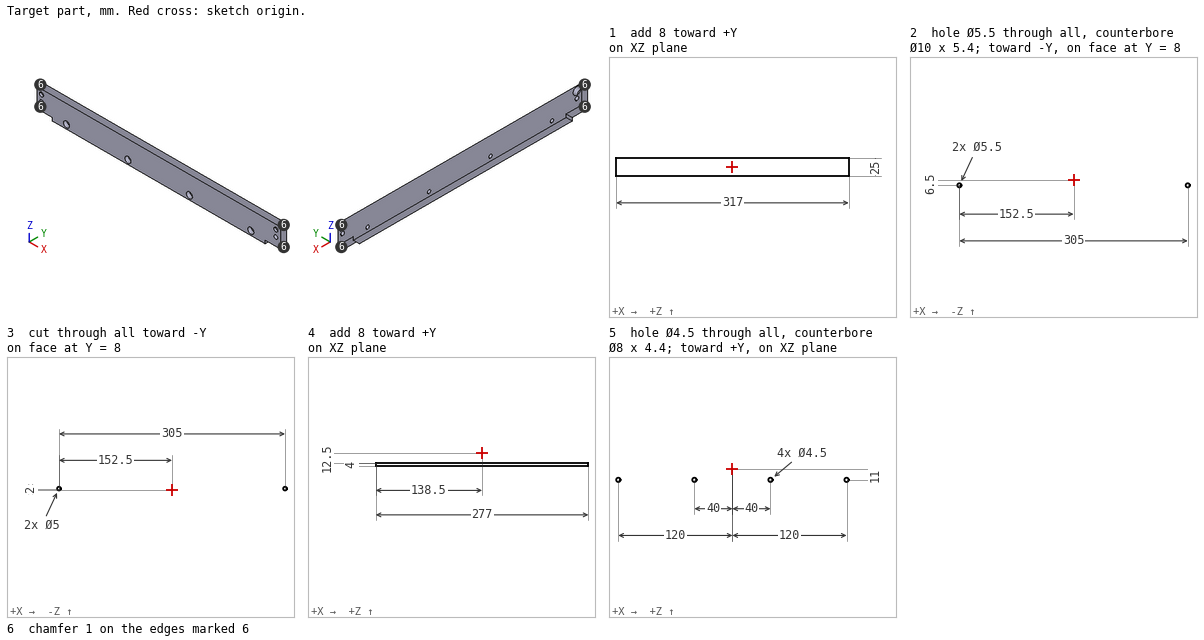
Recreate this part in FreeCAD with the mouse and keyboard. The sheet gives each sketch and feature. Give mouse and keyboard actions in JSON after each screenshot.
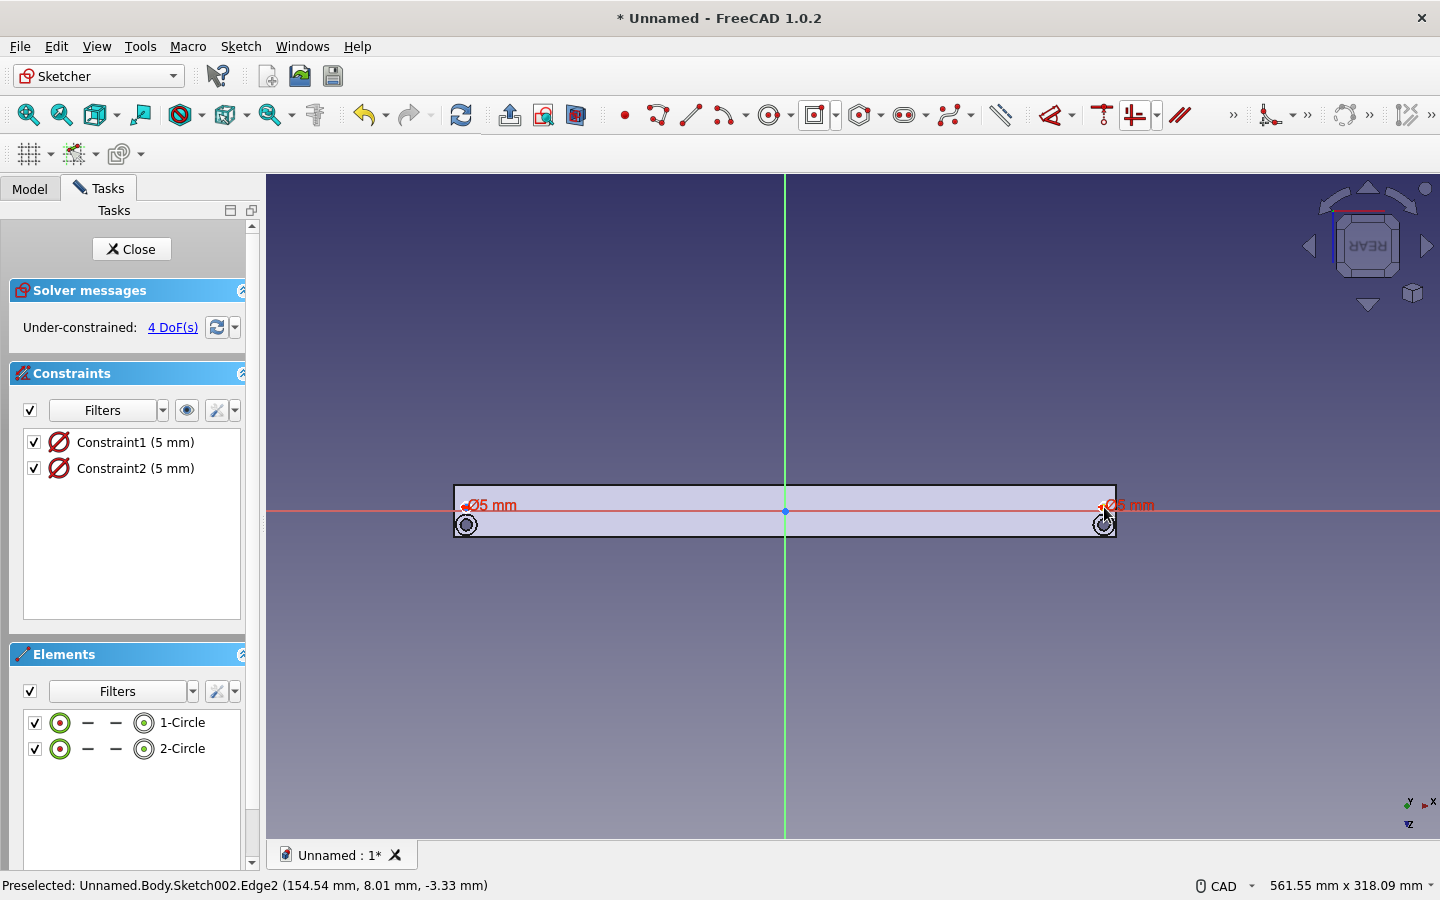
{"action": "left_click", "coordinate": [466, 507]}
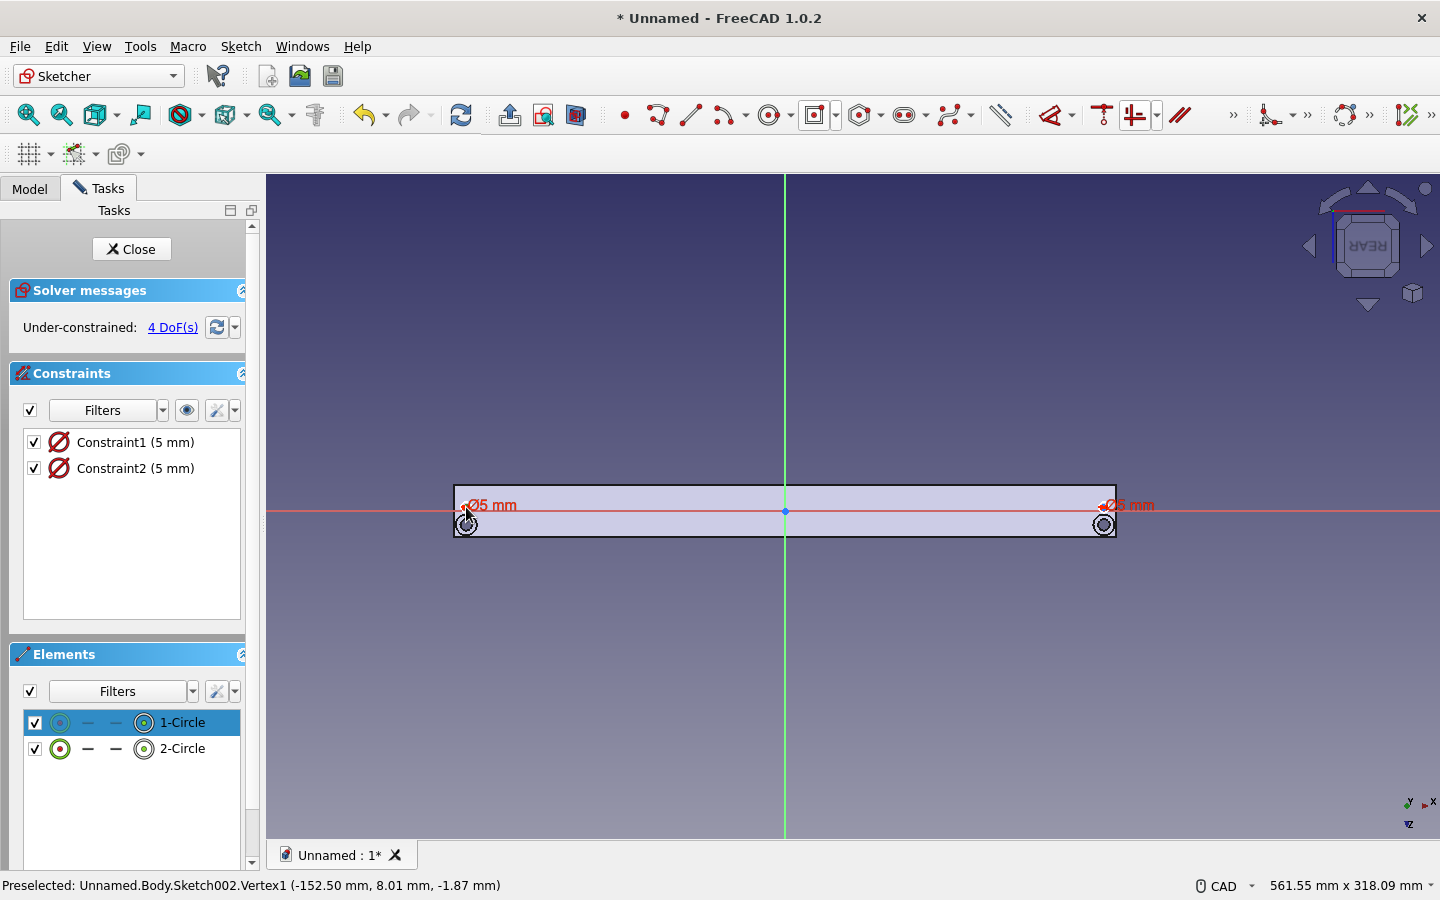
{"action": "left_click", "coordinate": [1104, 507]}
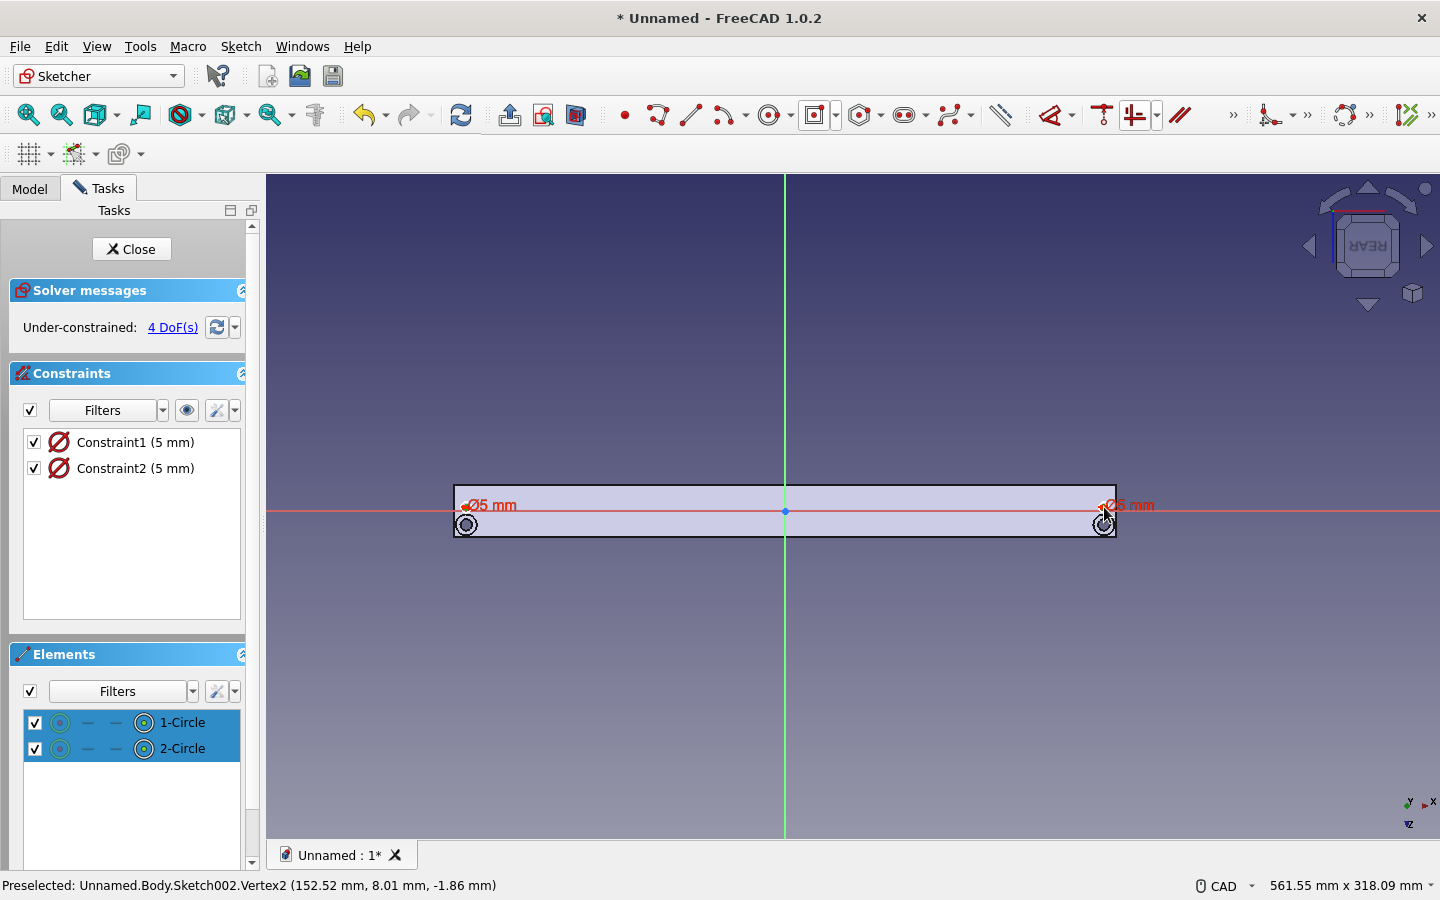
{"action": "key", "text": "h"}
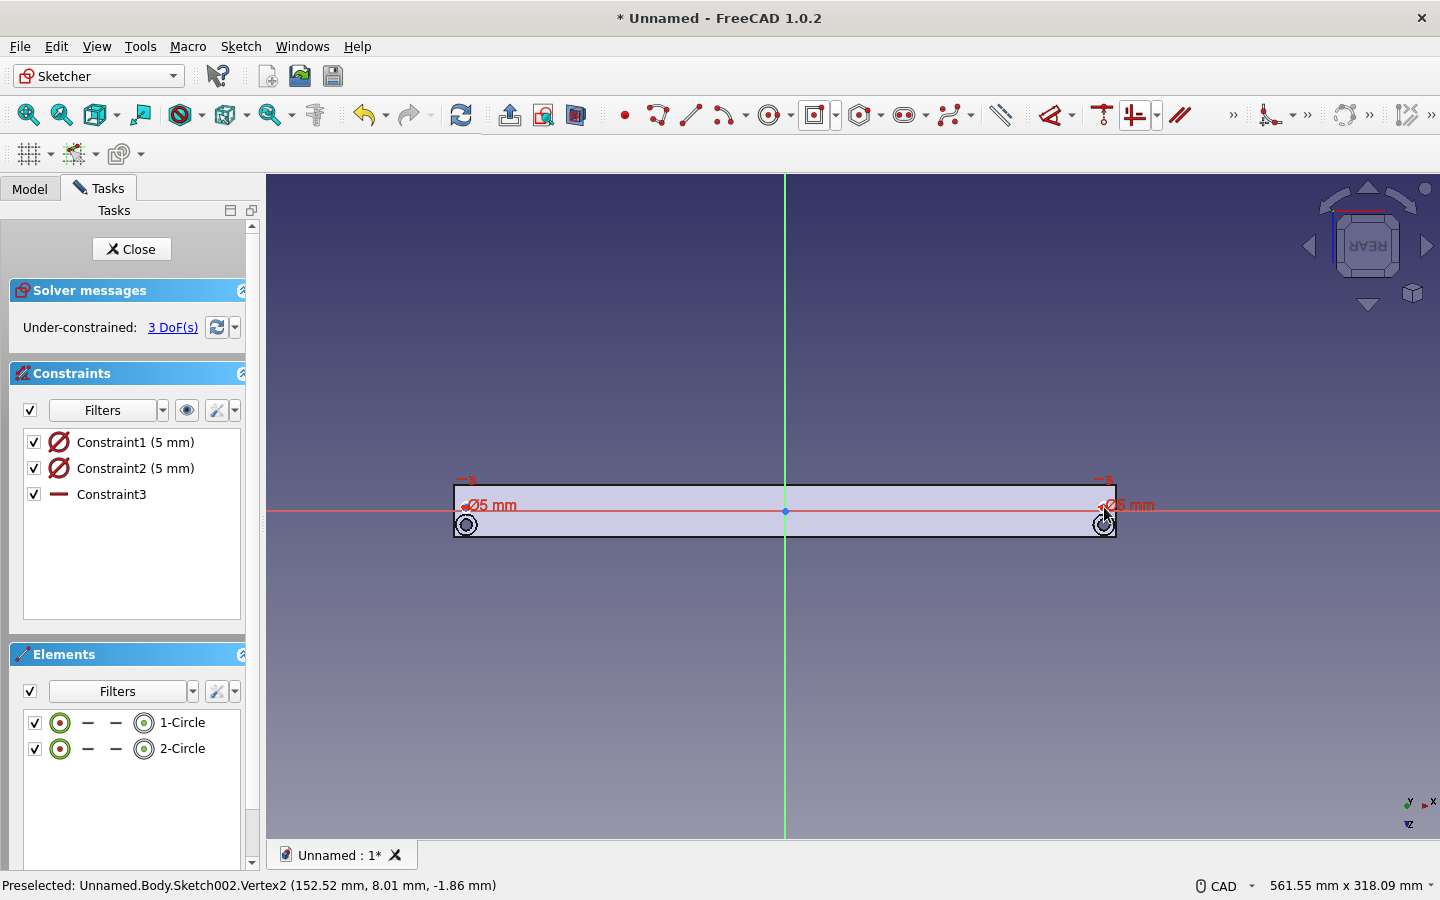
{"action": "left_click", "coordinate": [1050, 116]}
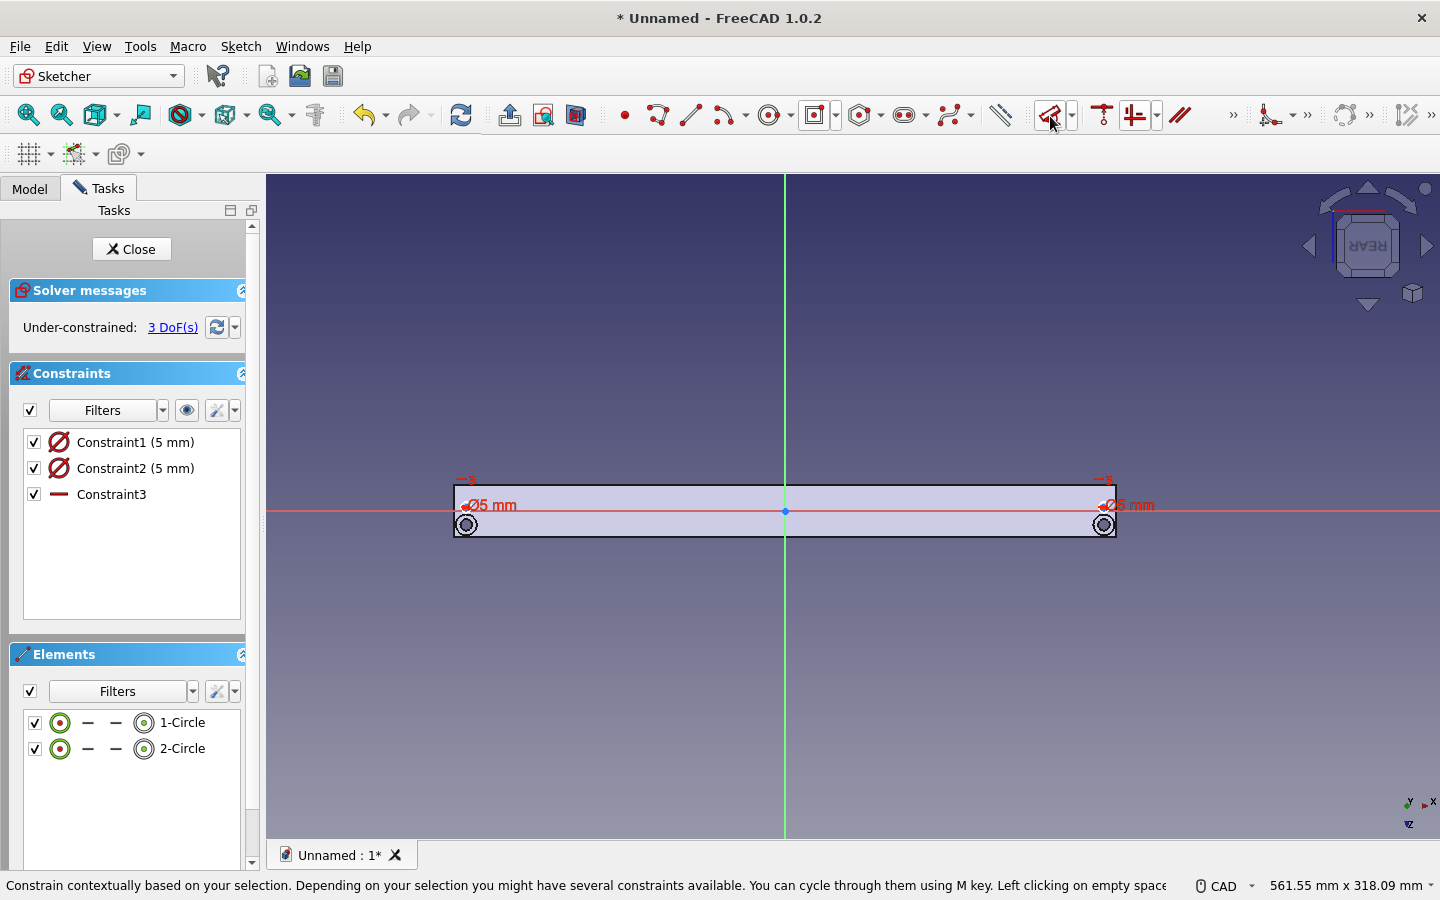
{"action": "scroll", "coordinate": [466, 507], "scroll_direction": "up", "scroll_amount": 12}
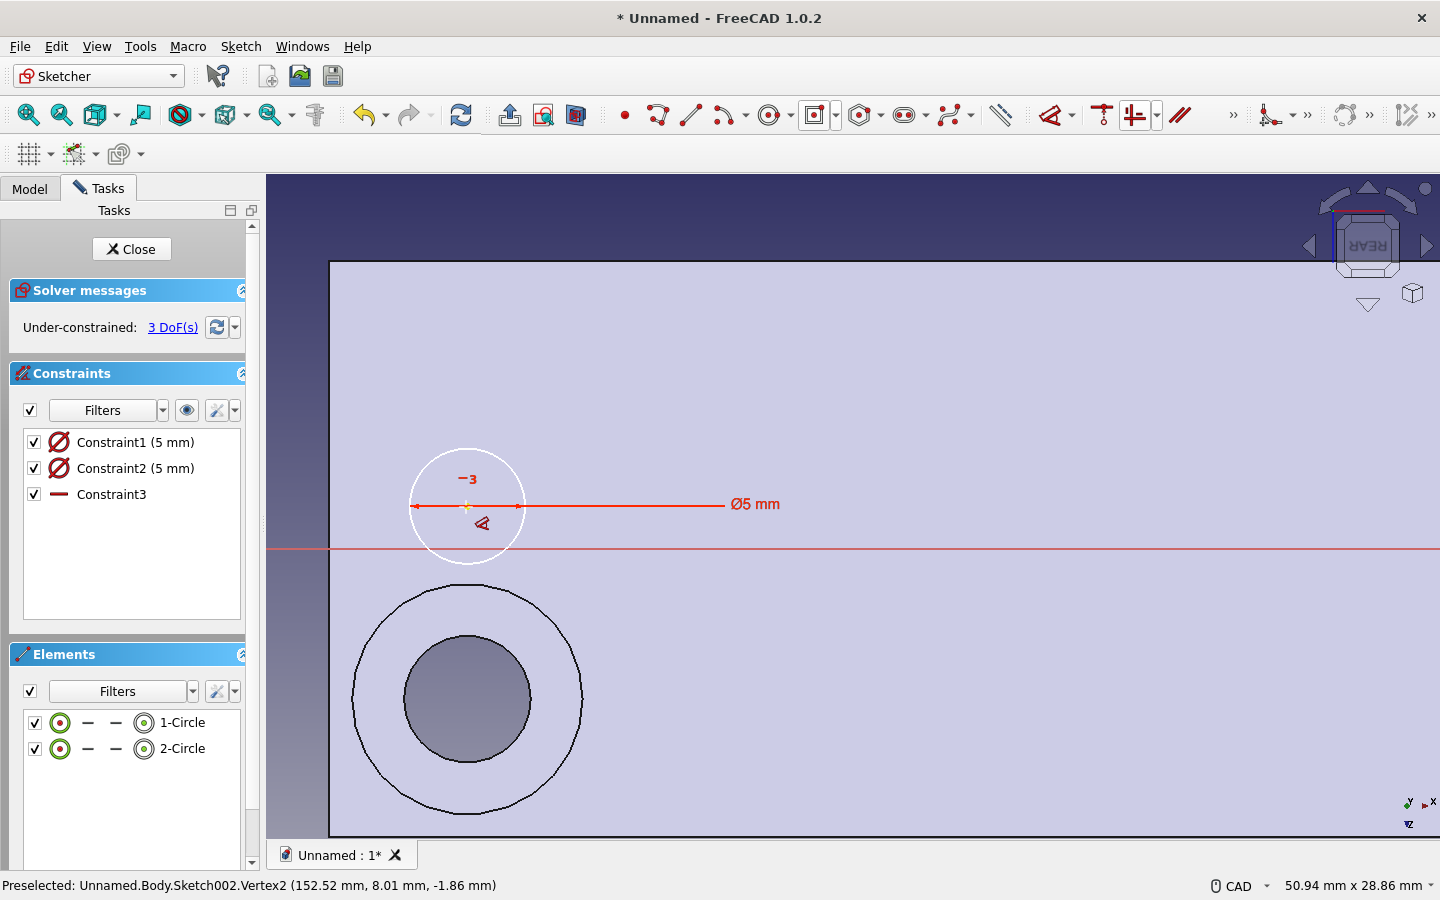
{"action": "left_click", "coordinate": [467, 506]}
{"action": "left_click", "coordinate": [433, 528]}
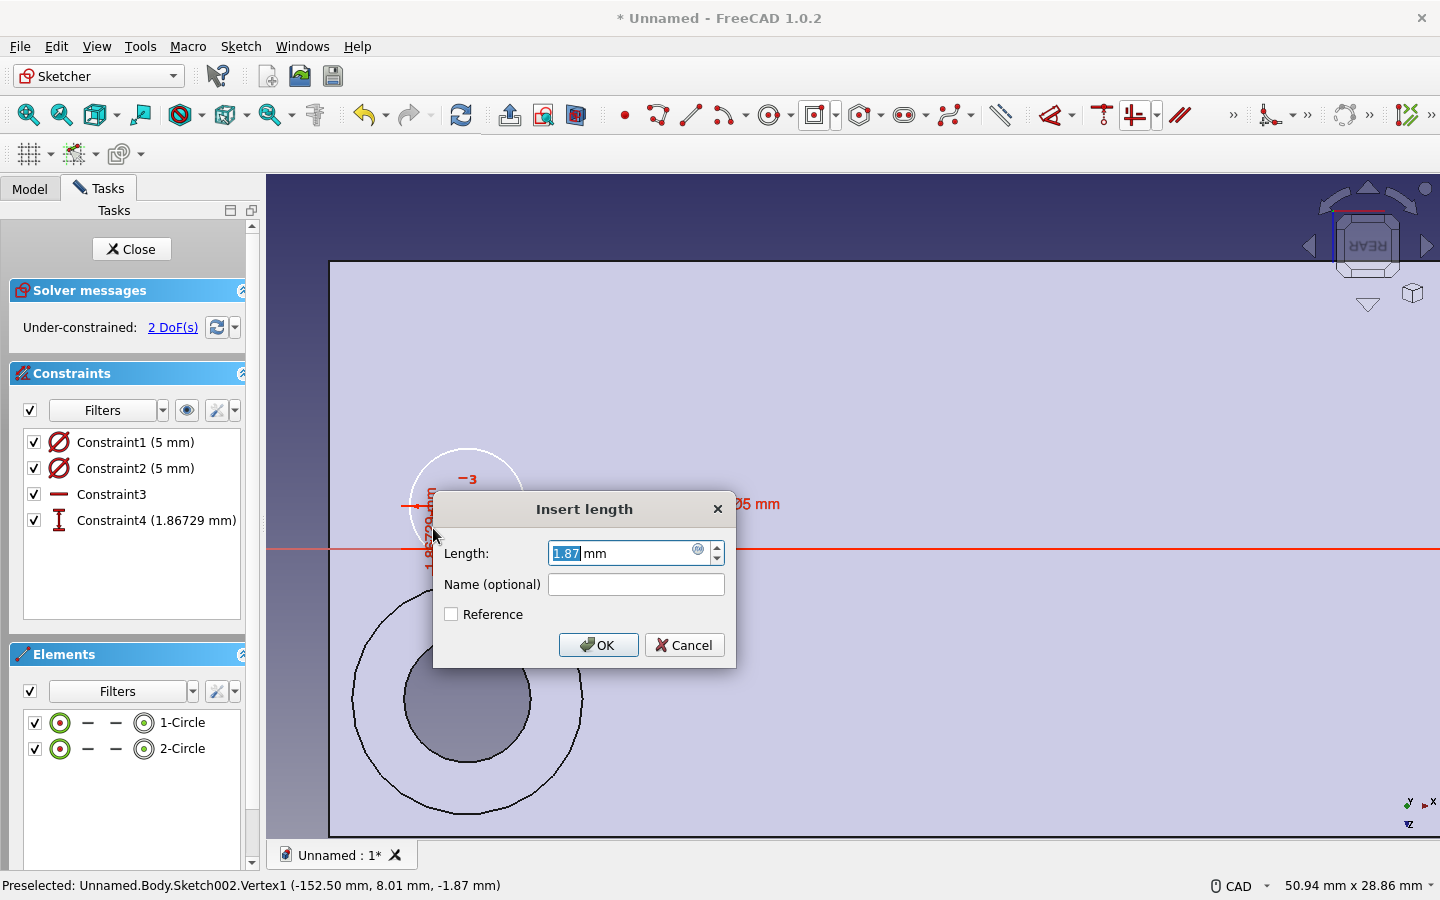
{"action": "type", "text": "2"}
{"action": "key", "text": "Return"}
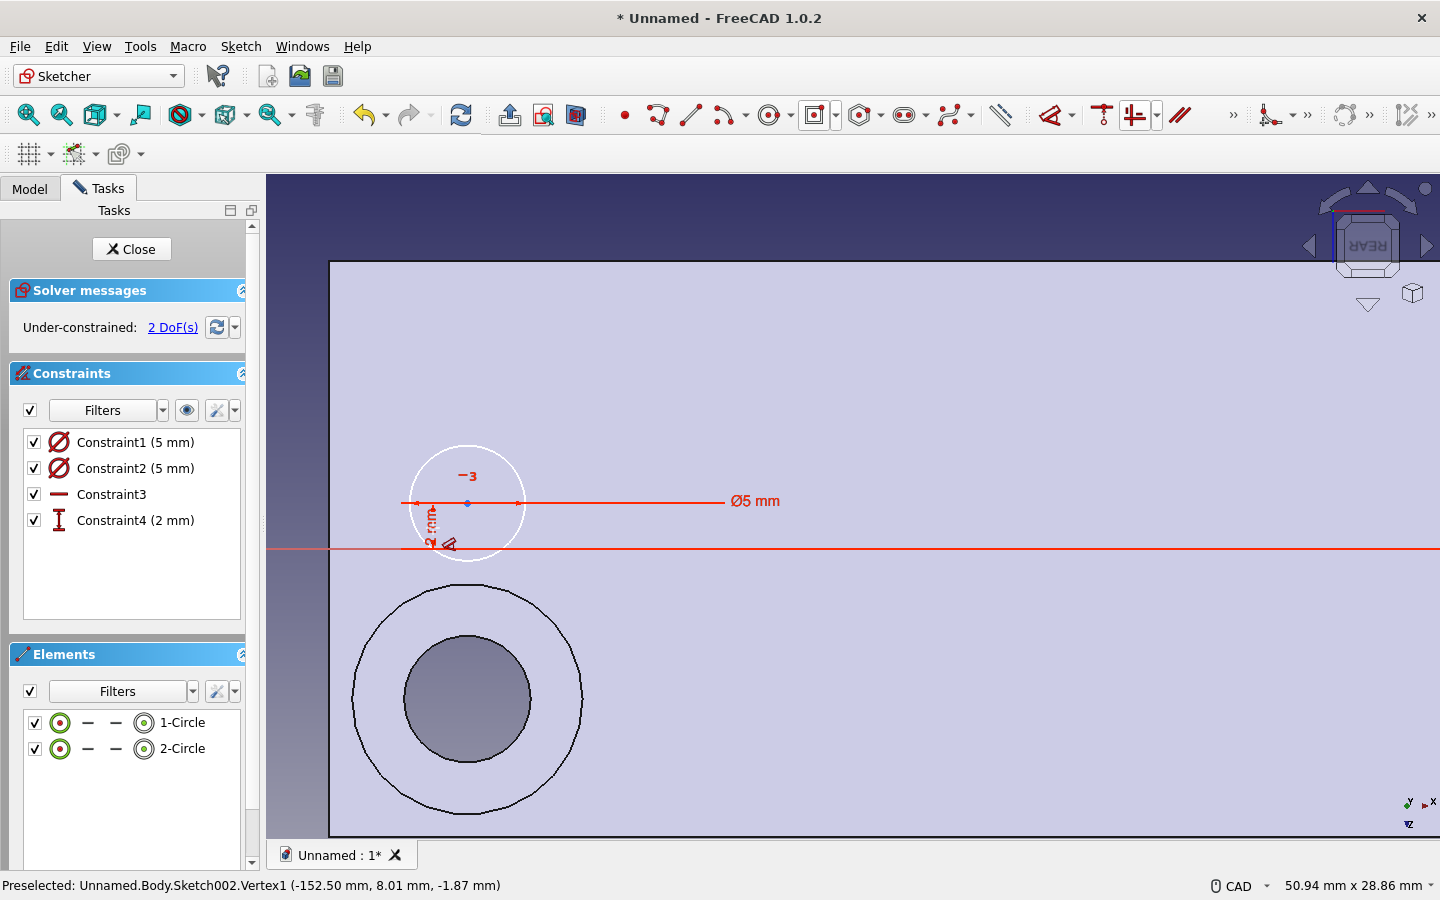
{"action": "scroll", "coordinate": [466, 507], "scroll_direction": "down", "scroll_amount": 12}